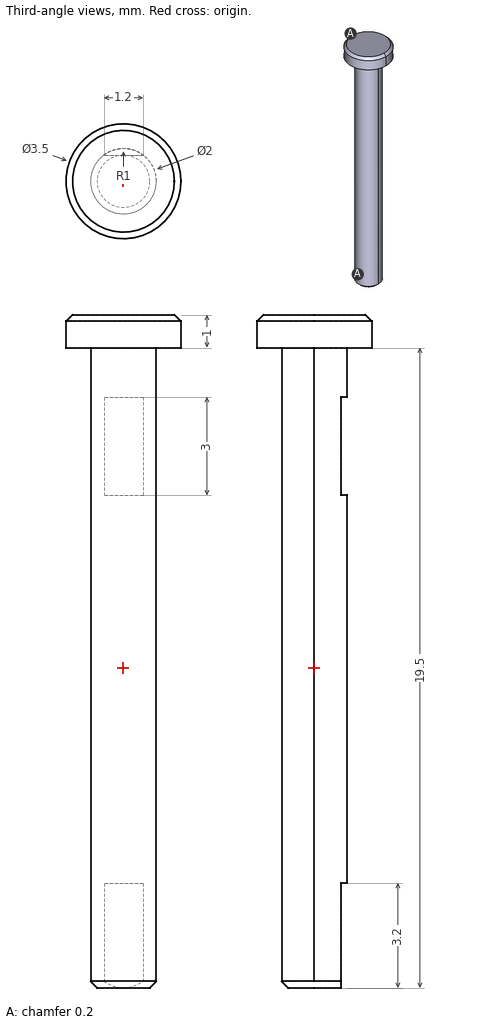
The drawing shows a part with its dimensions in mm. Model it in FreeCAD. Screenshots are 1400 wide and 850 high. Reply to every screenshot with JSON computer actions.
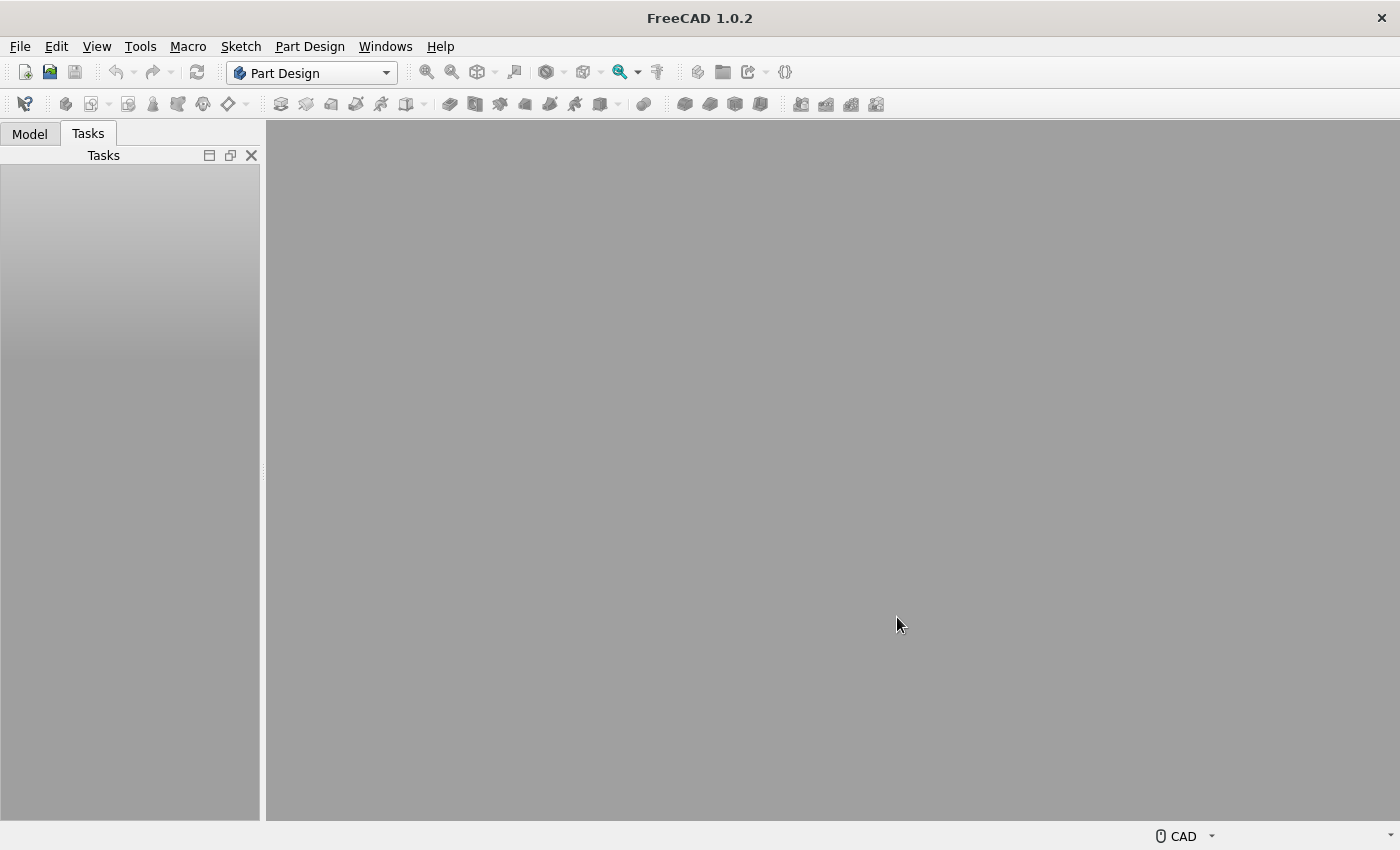
{"action": "key", "text": "ctrl+n"}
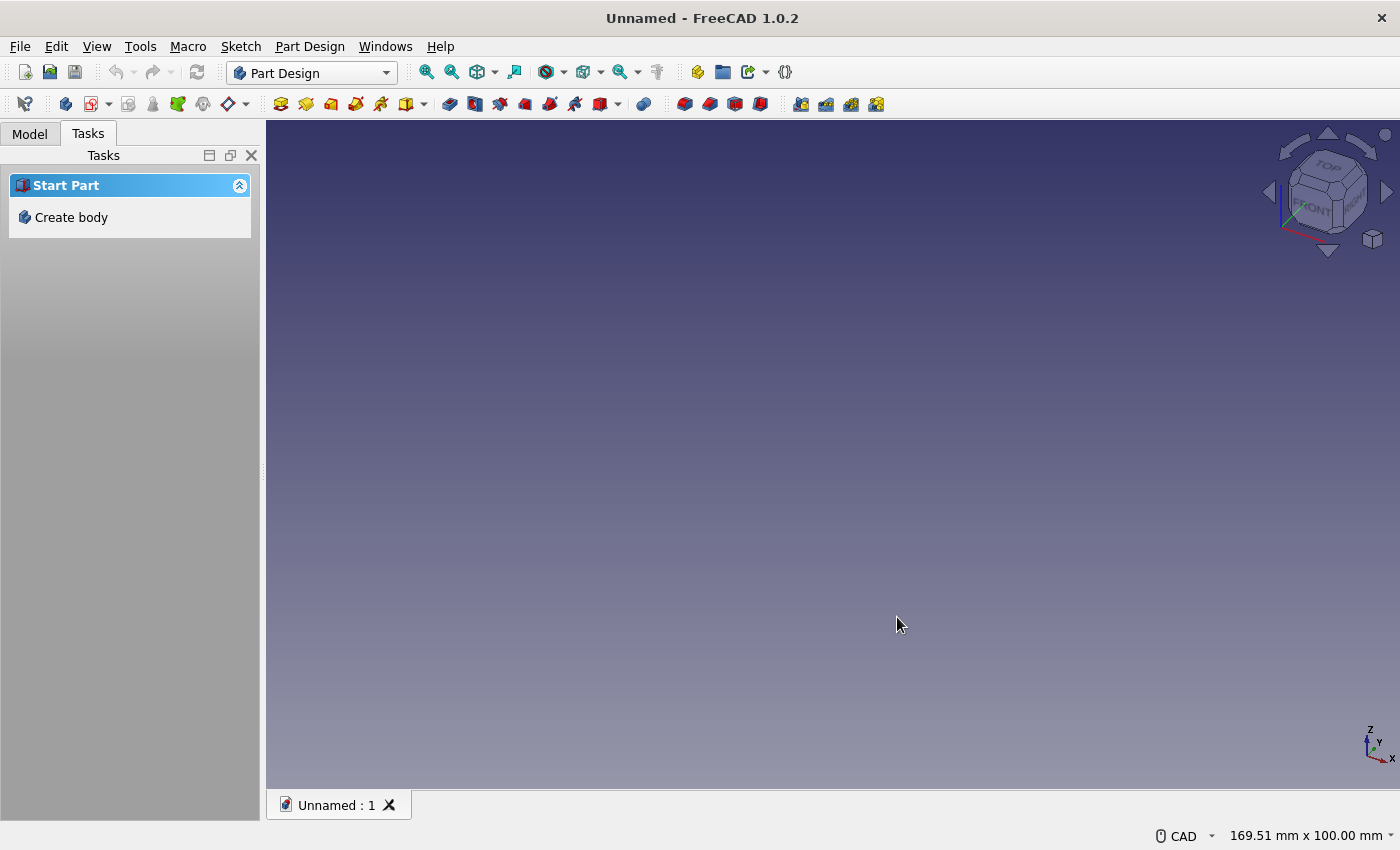
{"action": "left_click", "coordinate": [90, 104]}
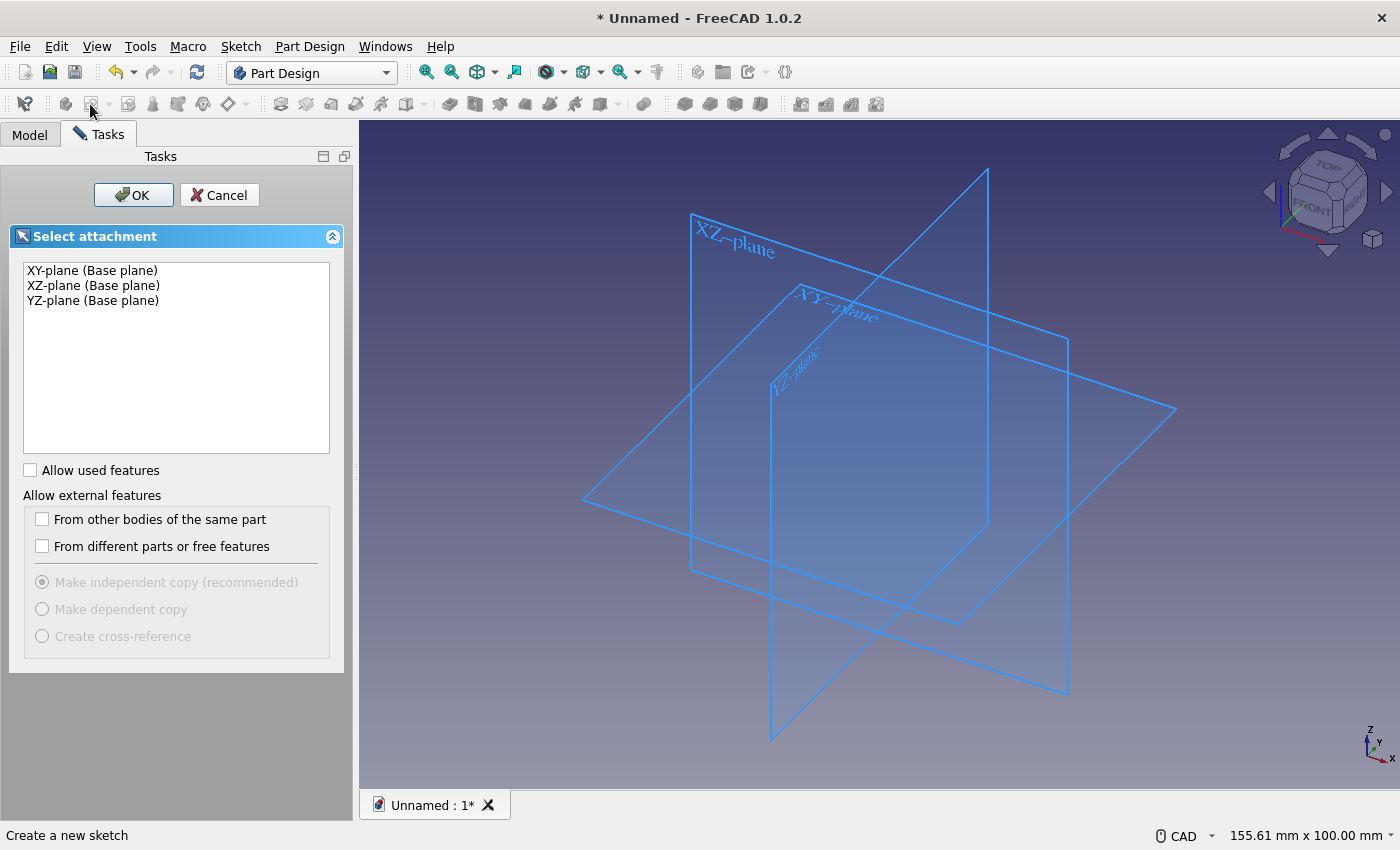
{"action": "left_click", "coordinate": [84, 270]}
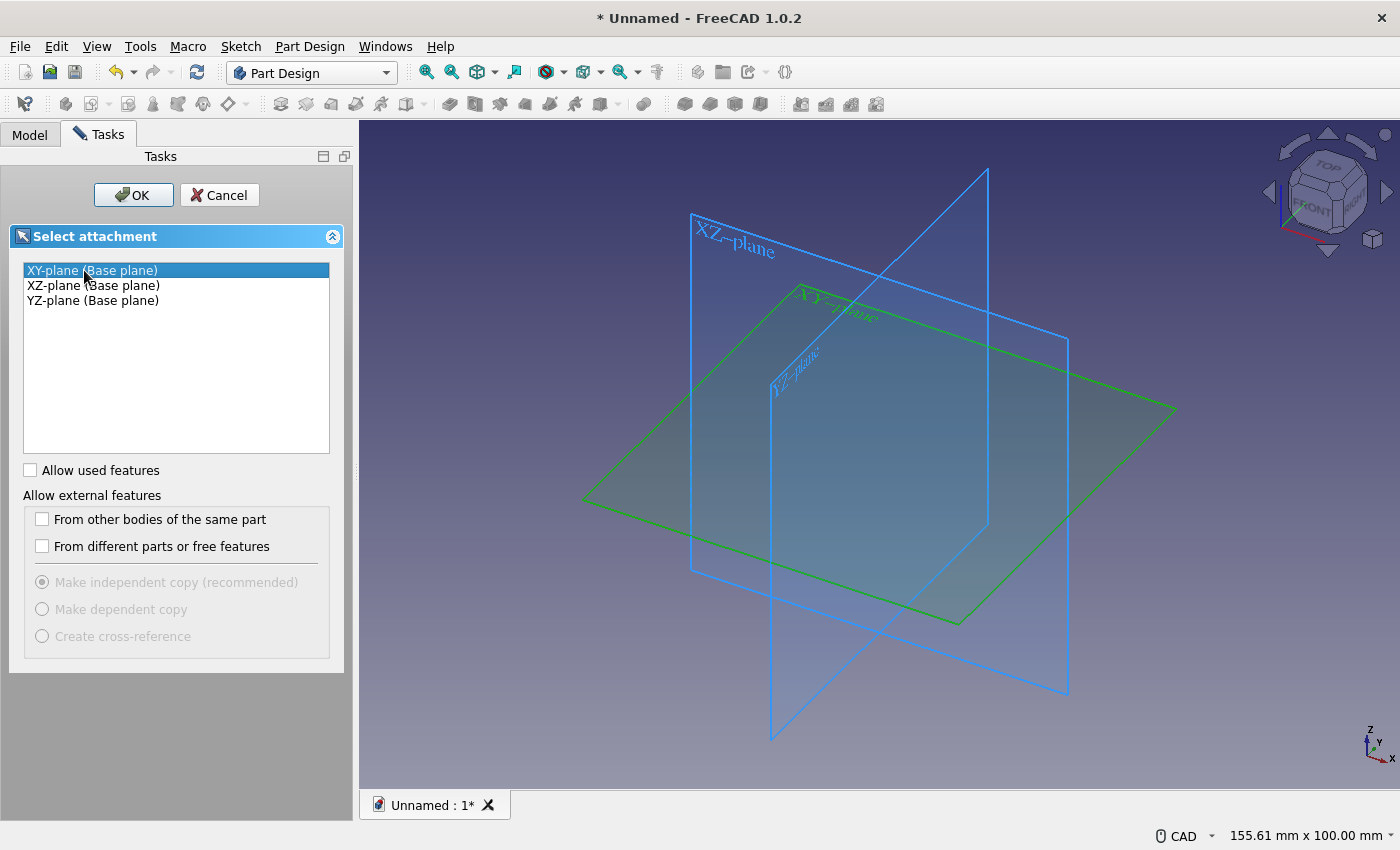
{"action": "left_click", "coordinate": [134, 195]}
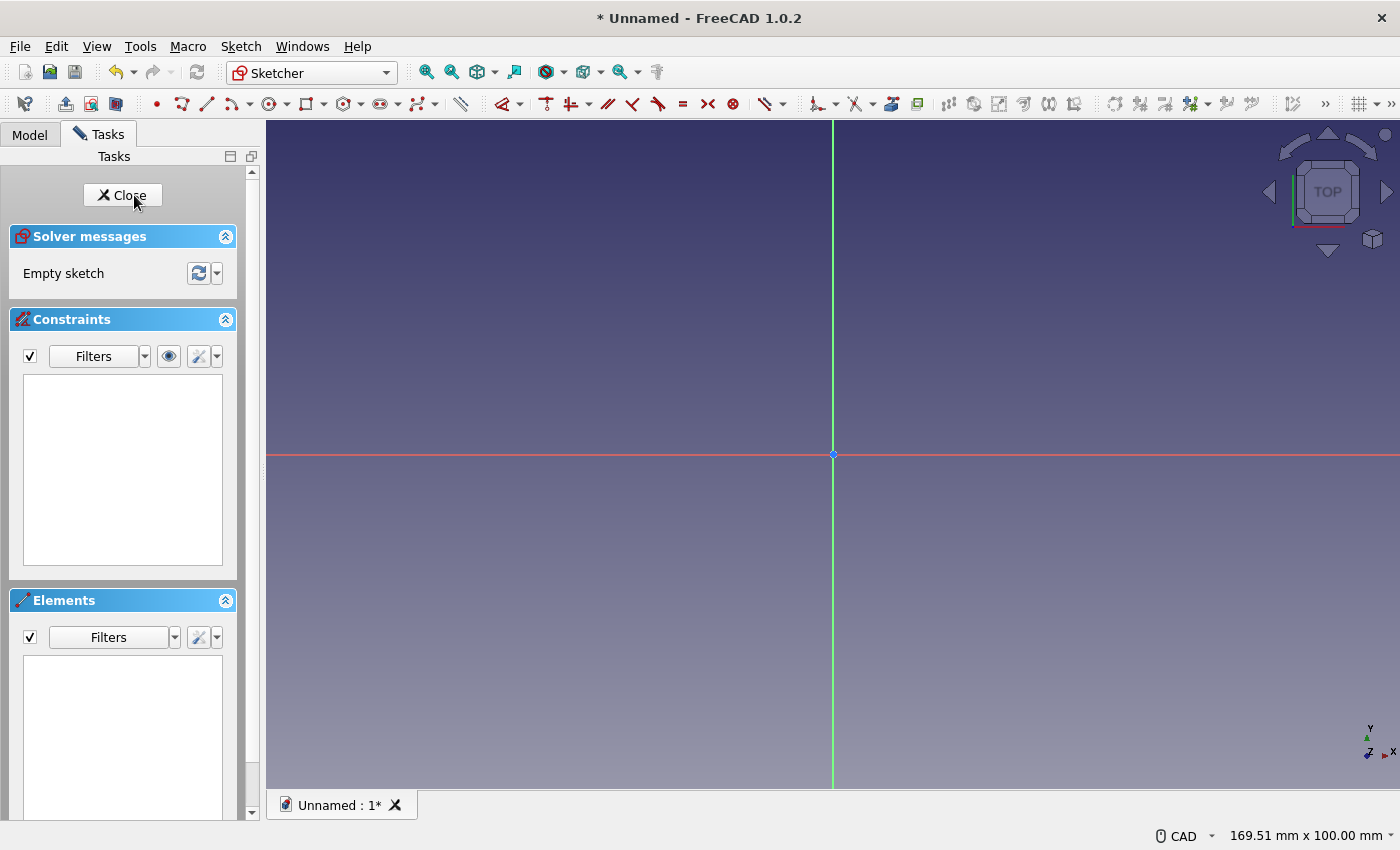
{"action": "scroll", "coordinate": [837, 455], "scroll_direction": "up", "scroll_amount": 15}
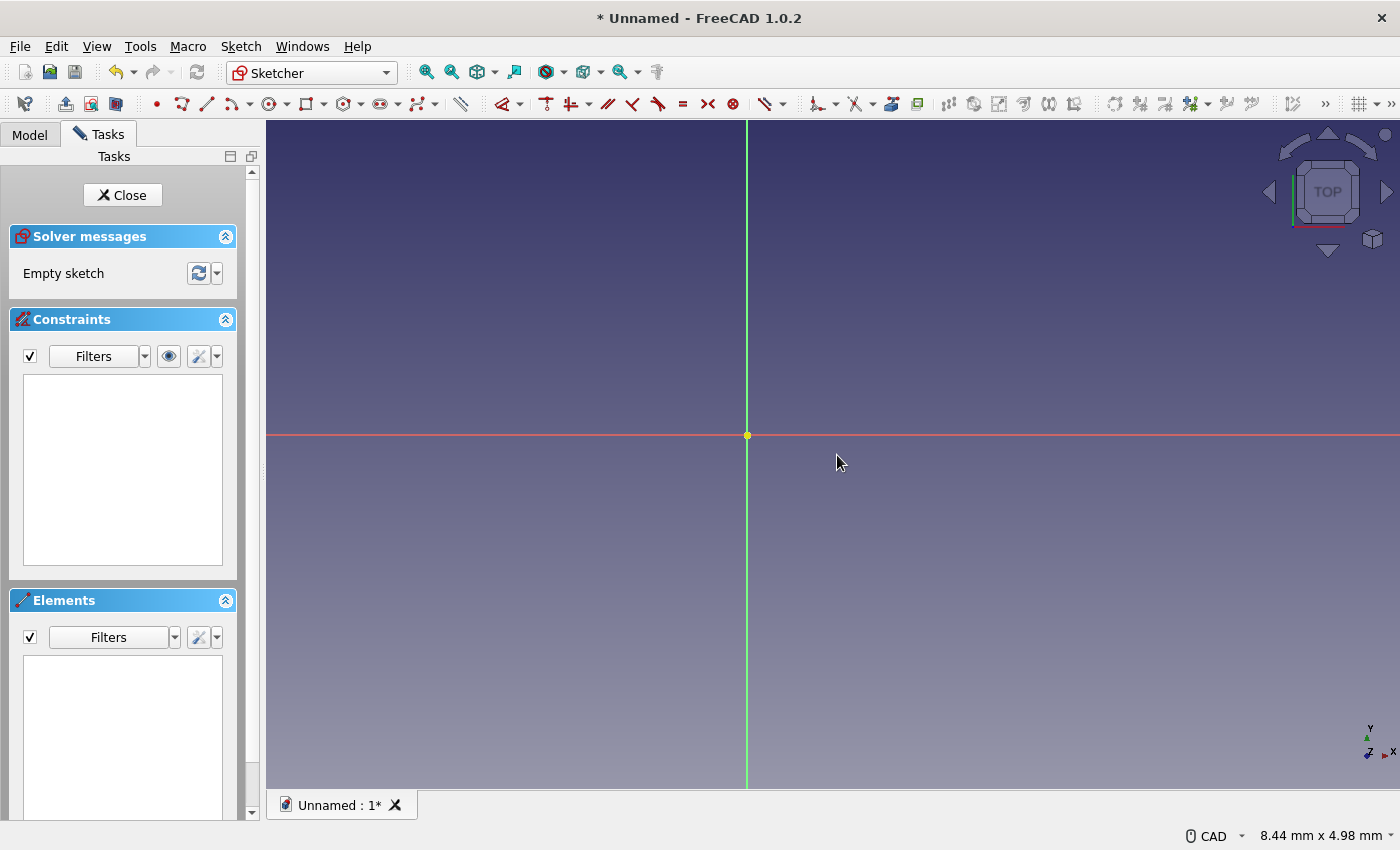
{"action": "scroll", "coordinate": [712, 397], "scroll_direction": "up", "scroll_amount": 2}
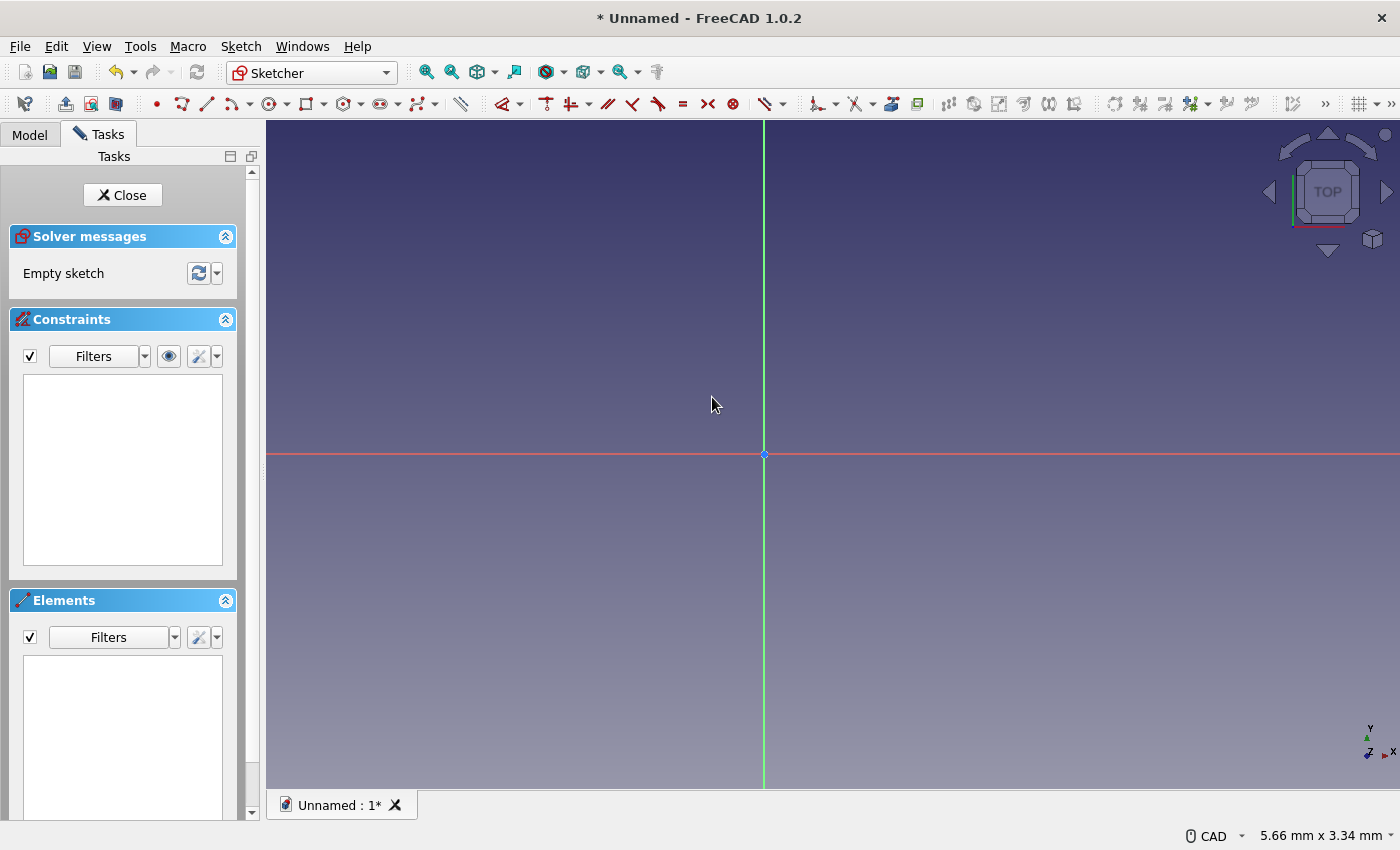
{"action": "key", "text": "g c"}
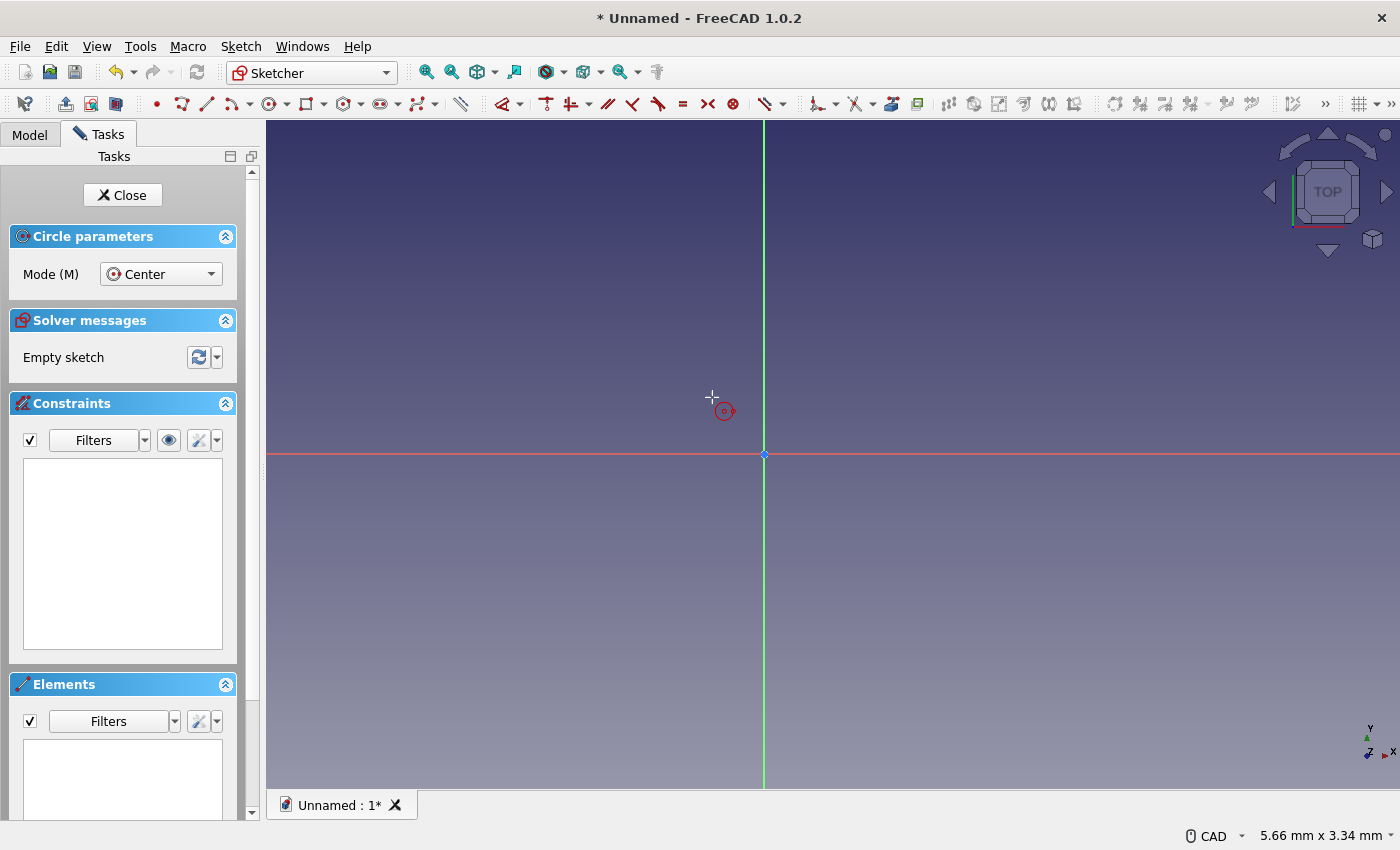
{"action": "left_click", "coordinate": [764, 454]}
{"action": "mouse_move", "coordinate": [906, 312]}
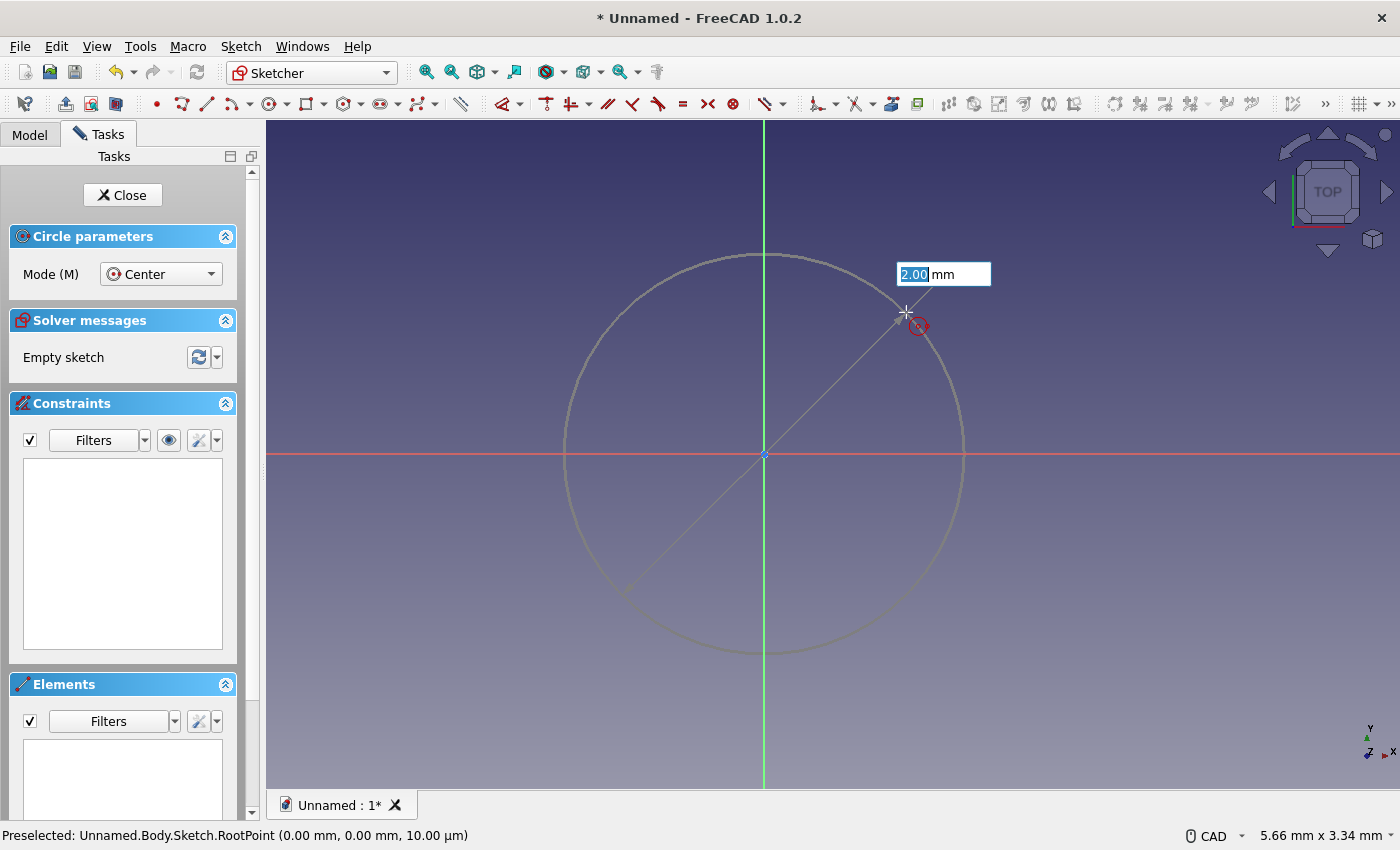
{"action": "type", "text": "2"}
{"action": "key", "text": "Return"}
{"action": "key", "text": "Escape"}